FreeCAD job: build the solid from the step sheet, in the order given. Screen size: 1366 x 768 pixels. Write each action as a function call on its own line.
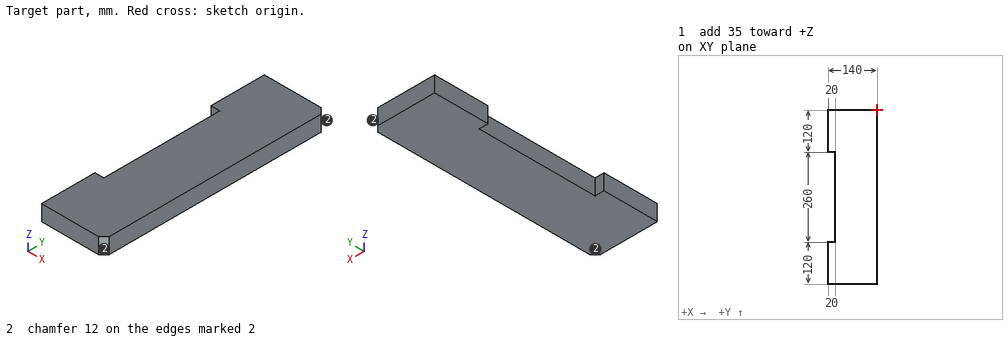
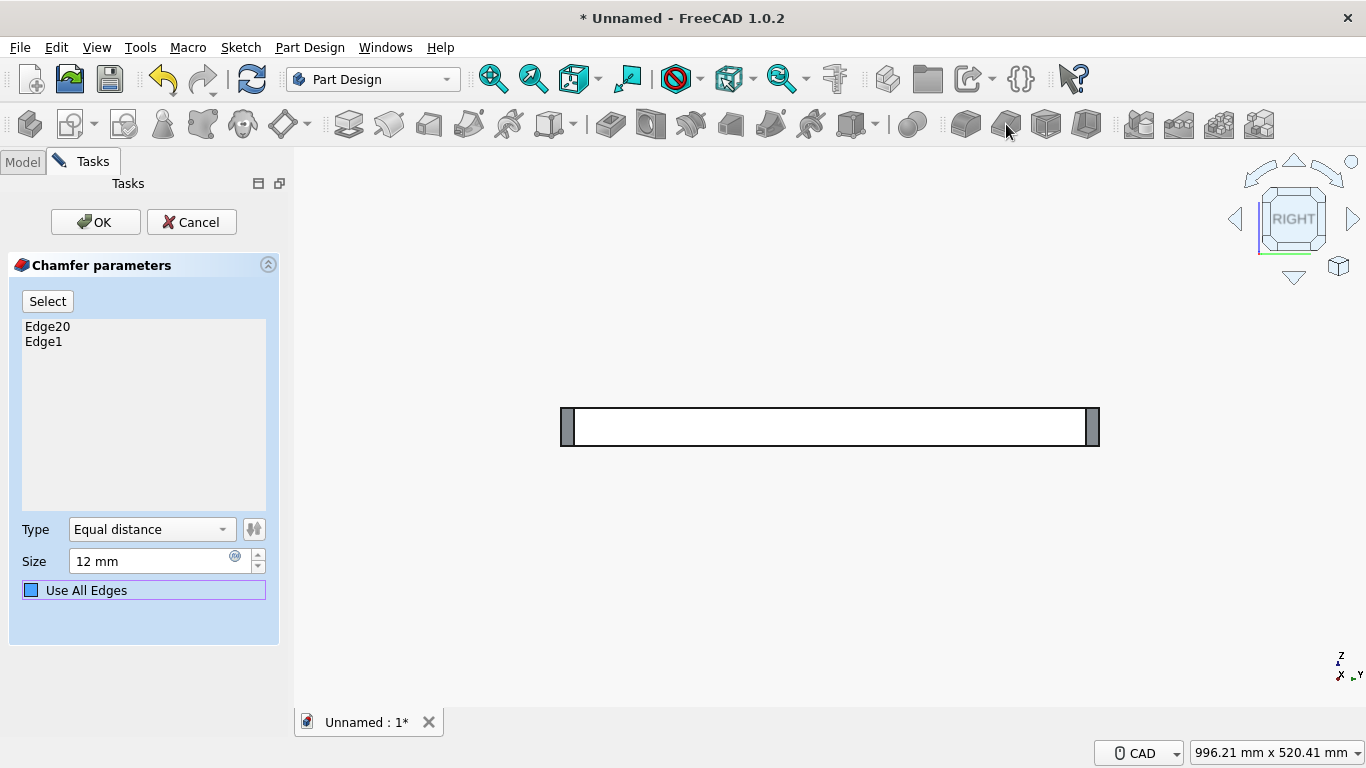
click(96, 222)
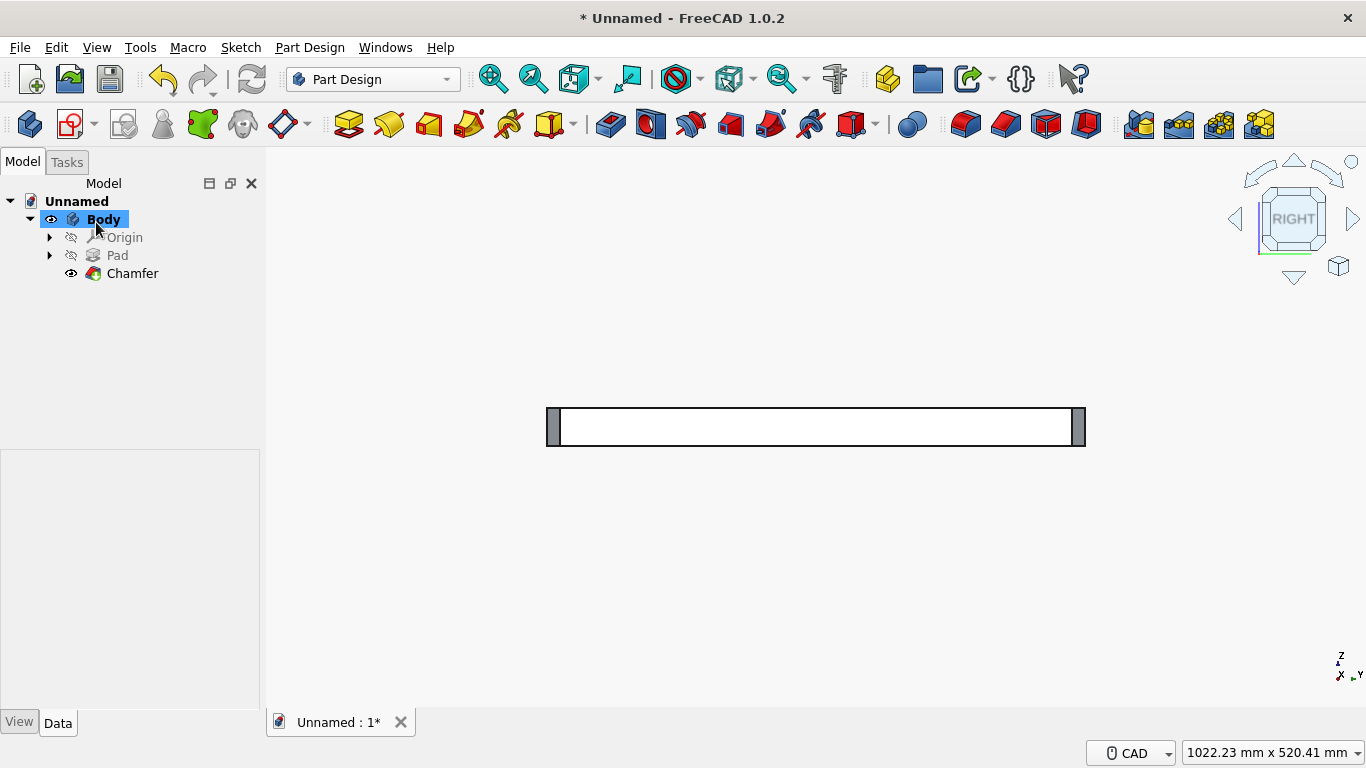
key(0)